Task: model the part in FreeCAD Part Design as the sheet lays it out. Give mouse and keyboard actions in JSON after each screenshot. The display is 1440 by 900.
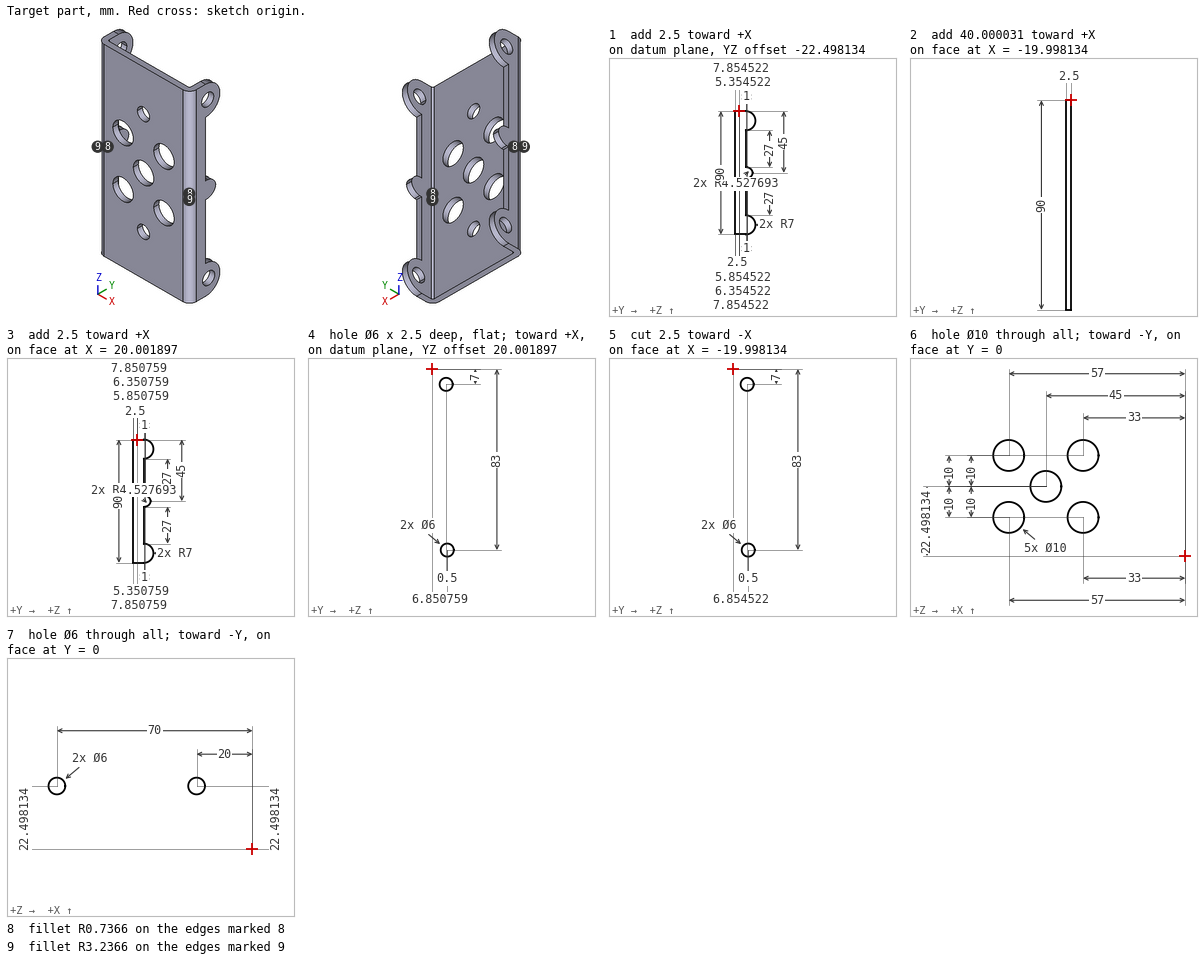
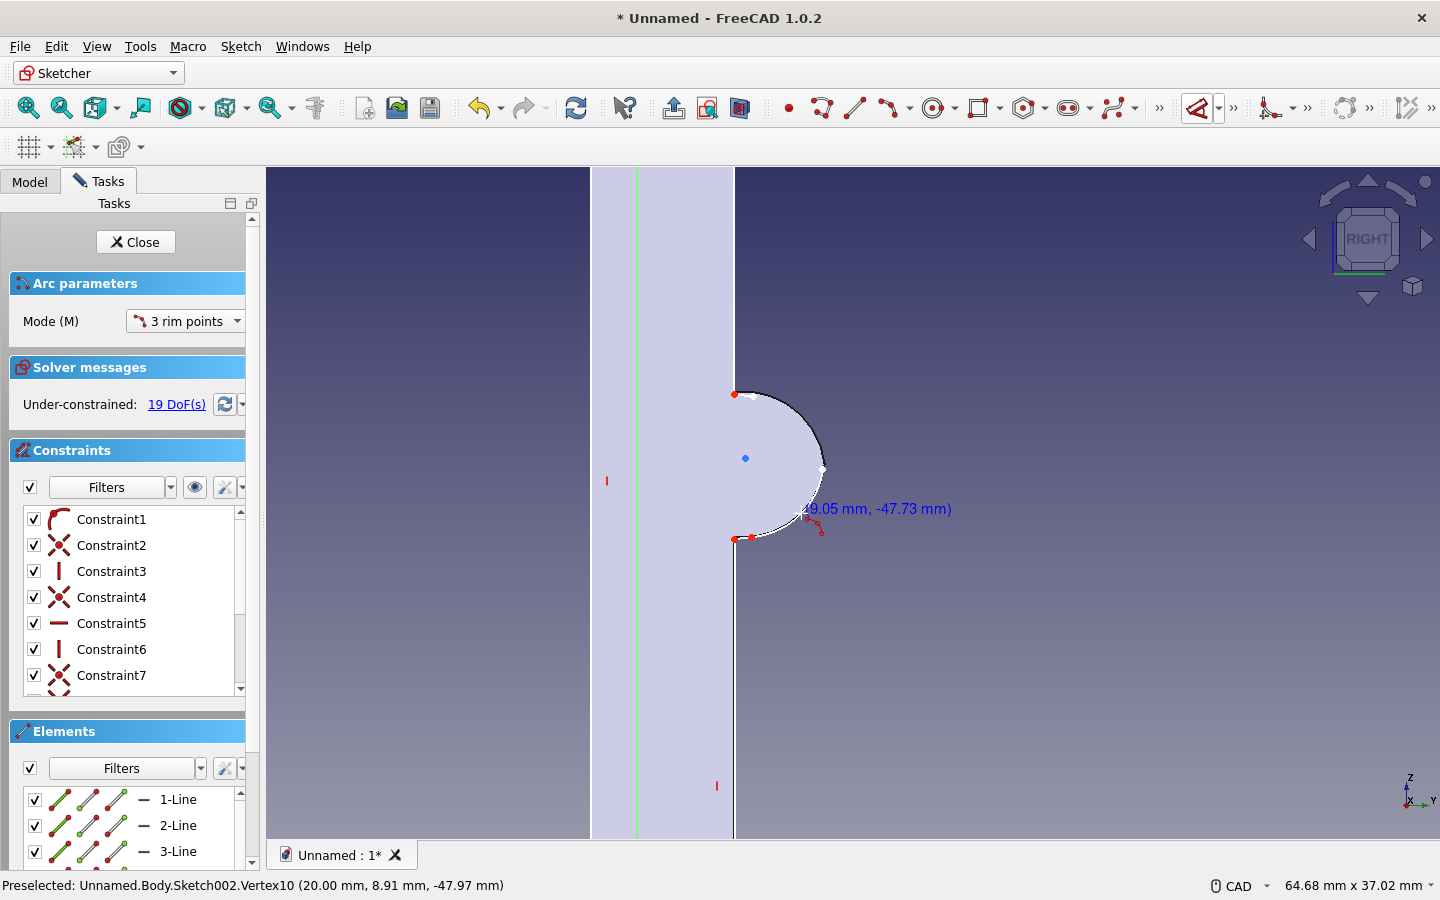
{"action": "scroll", "coordinate": [804, 516], "scroll_direction": "down", "scroll_amount": 7}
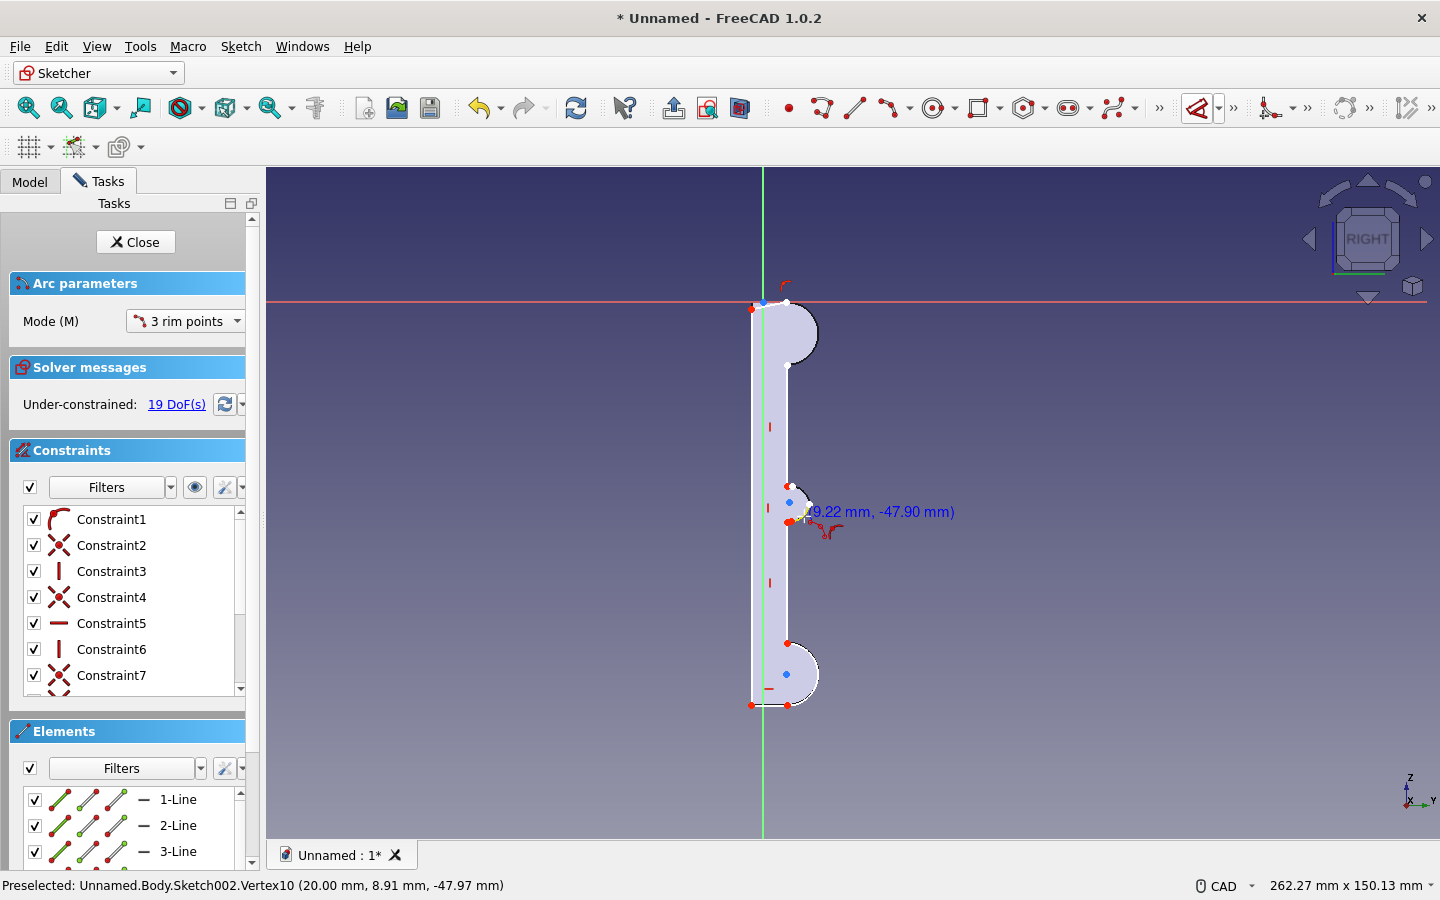
{"action": "left_click", "coordinate": [809, 505]}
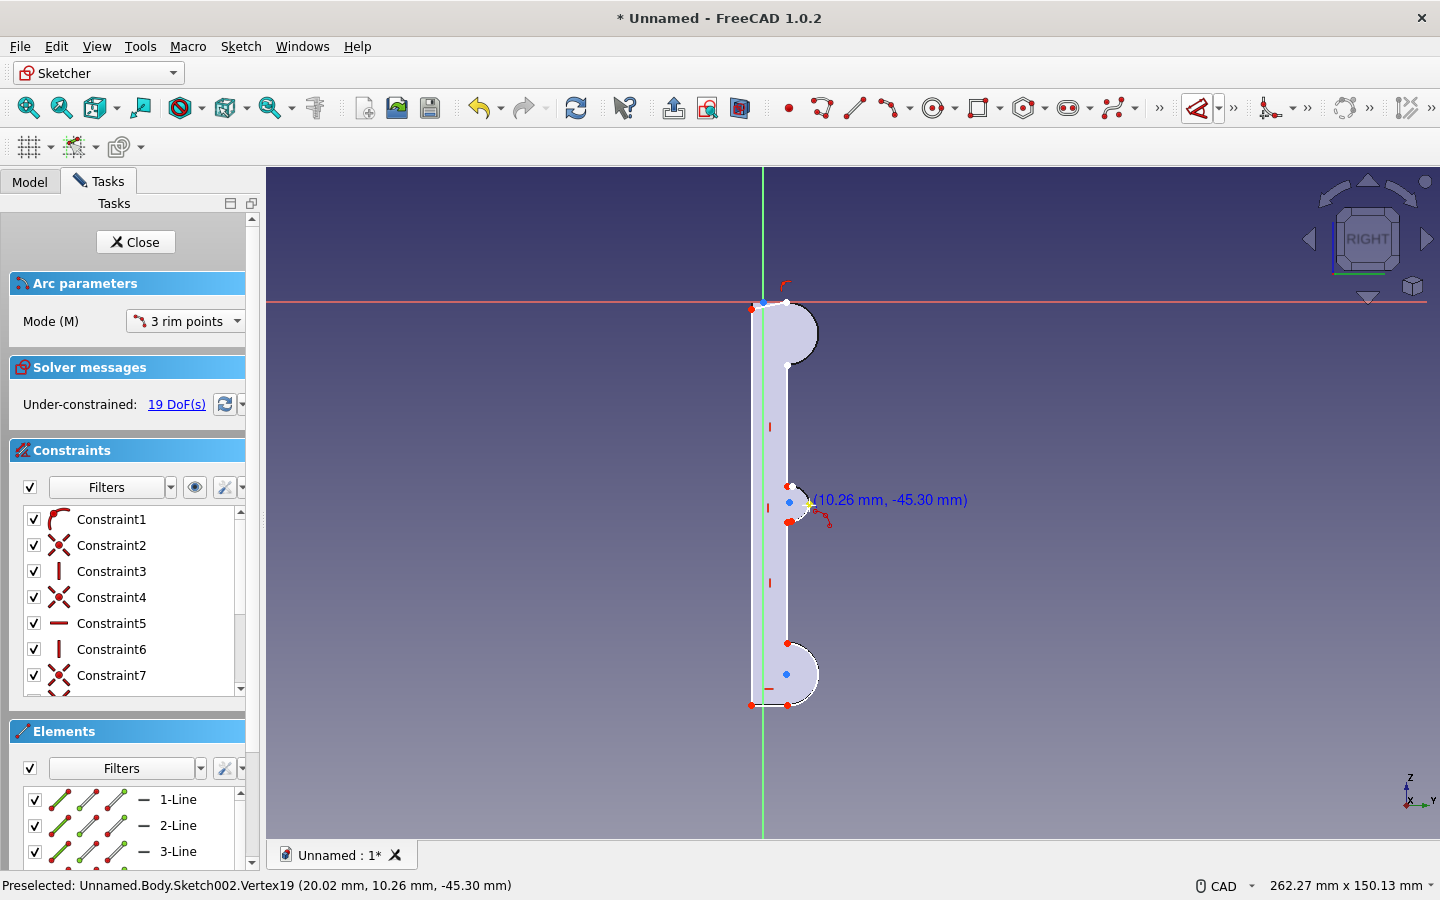
{"action": "scroll", "coordinate": [792, 486], "scroll_direction": "up", "scroll_amount": 10}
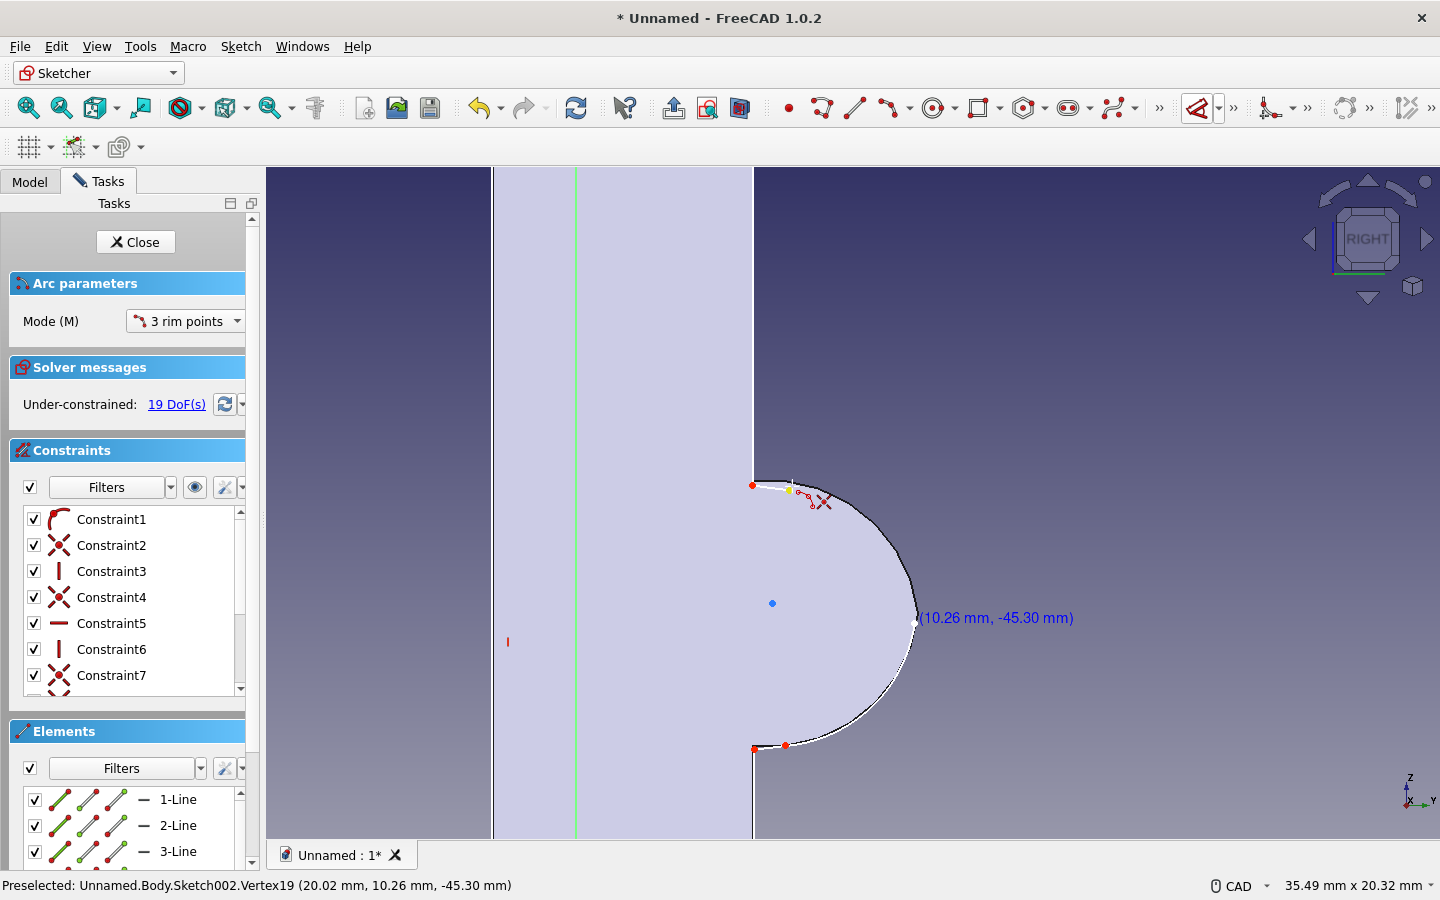
{"action": "left_click", "coordinate": [789, 490]}
{"action": "left_click", "coordinate": [875, 524]}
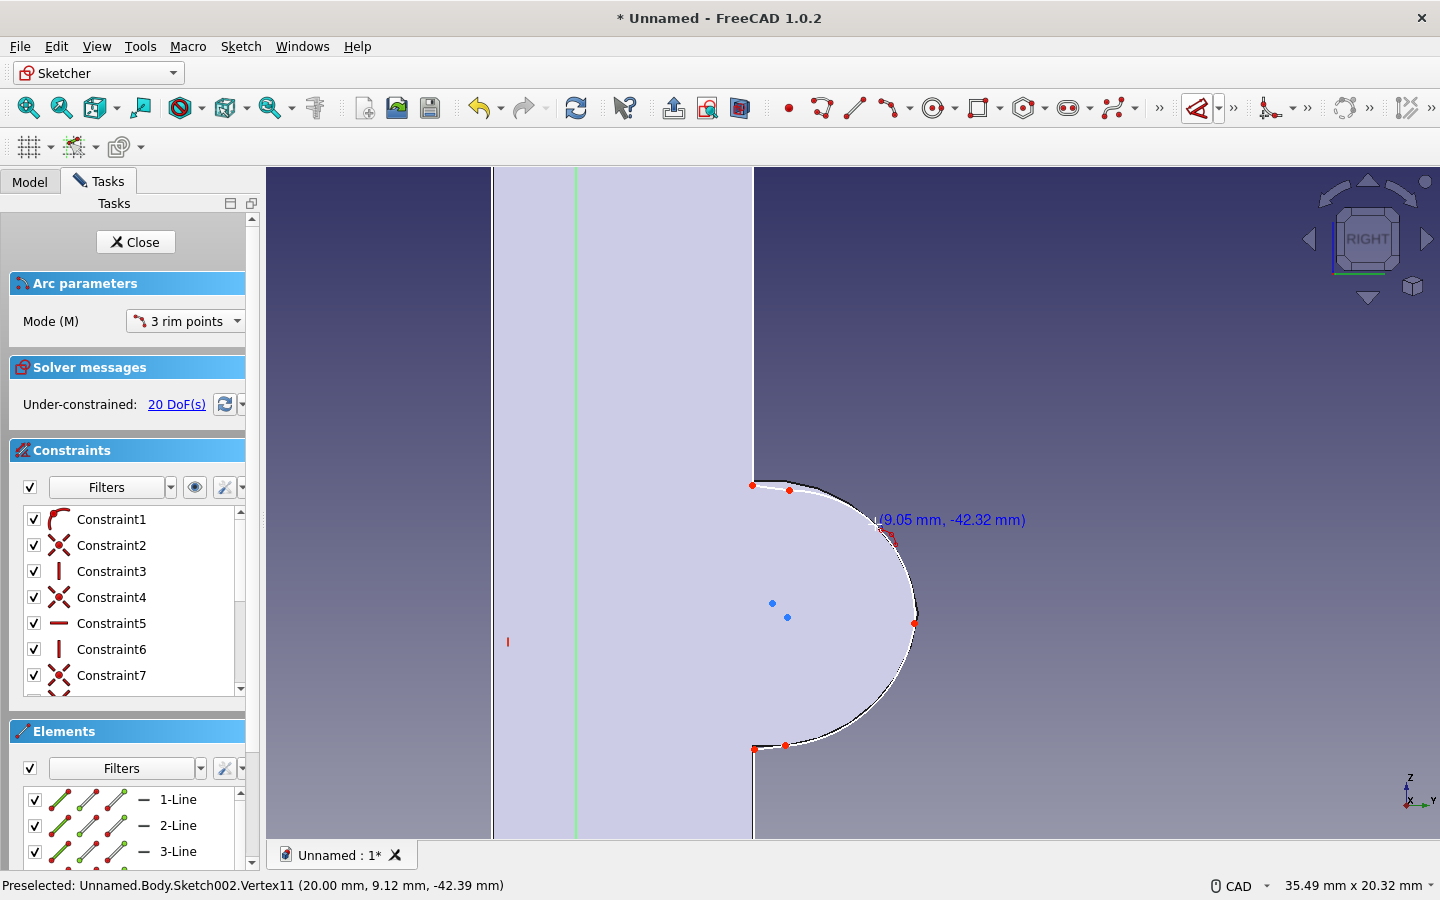
{"action": "scroll", "coordinate": [792, 486], "scroll_direction": "down", "scroll_amount": 10}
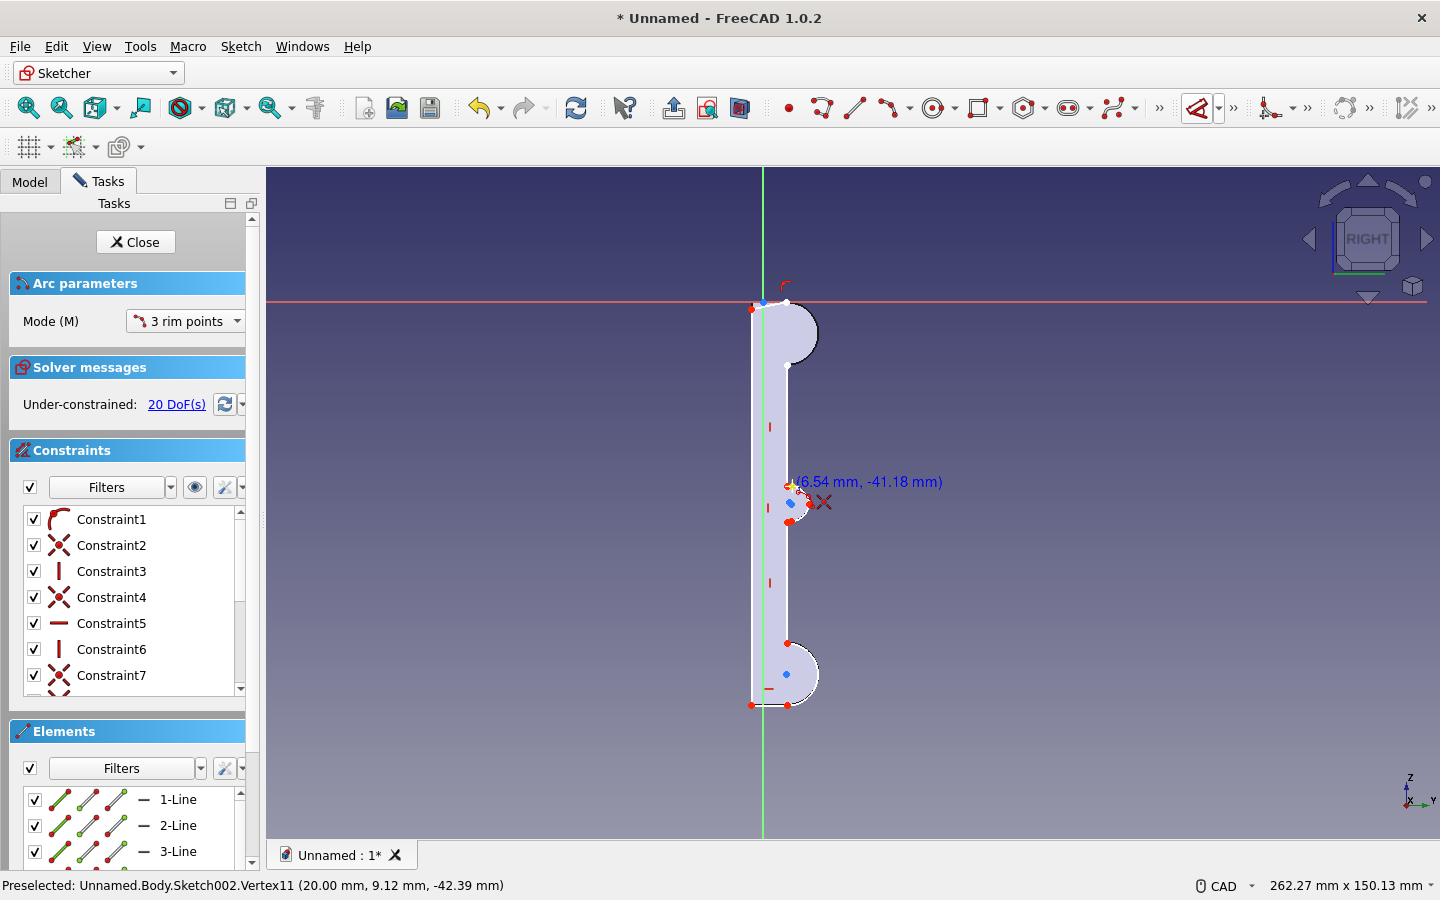
{"action": "left_click", "coordinate": [787, 366]}
{"action": "left_click", "coordinate": [787, 302]}
{"action": "left_click", "coordinate": [818, 334]}
{"action": "key", "text": "Escape"}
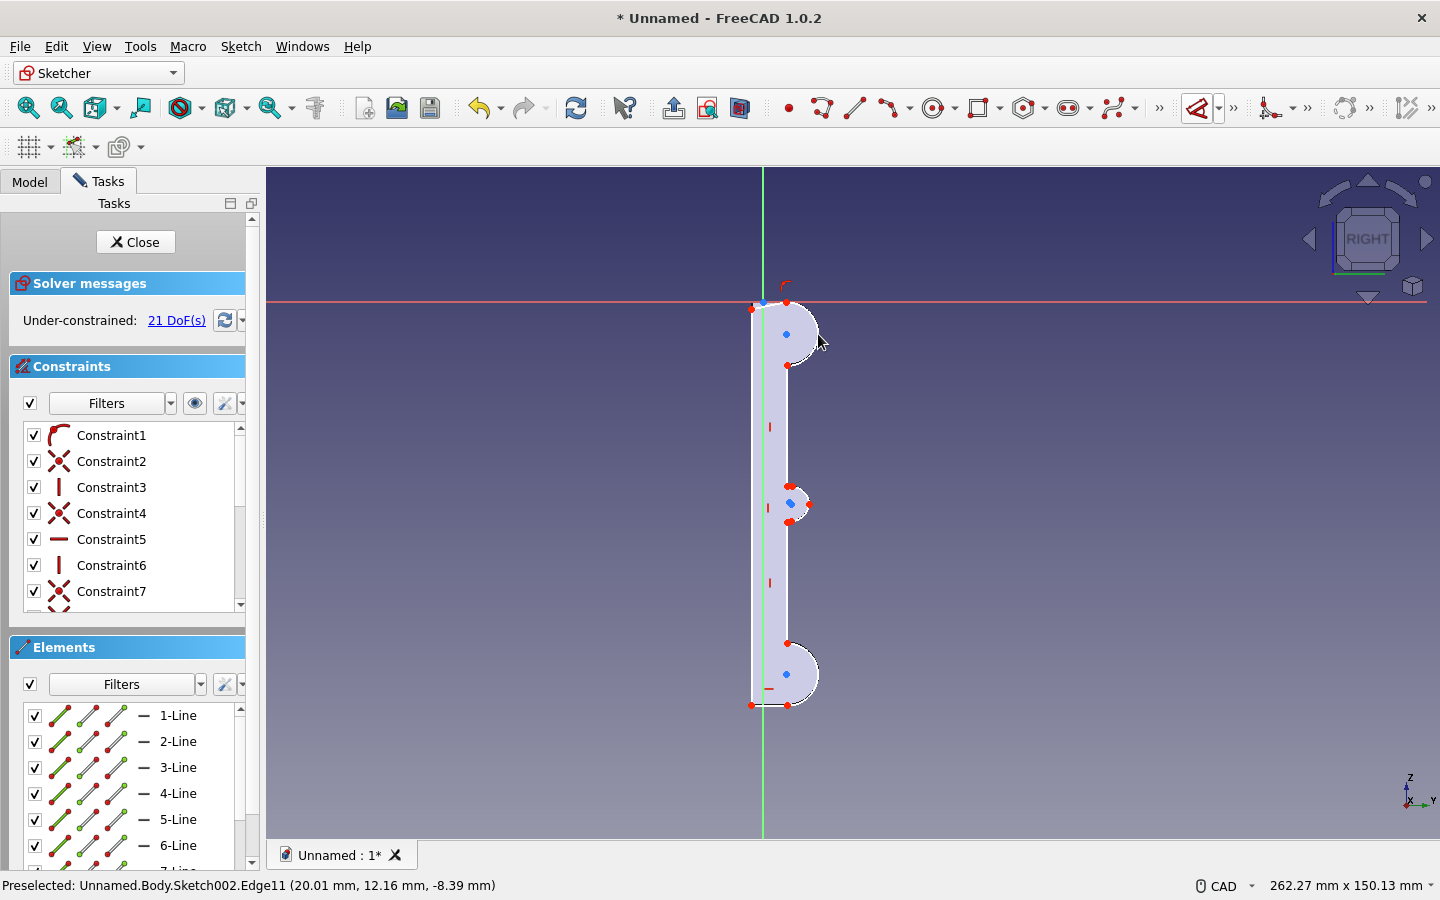
{"action": "scroll", "coordinate": [776, 304], "scroll_direction": "up", "scroll_amount": 2}